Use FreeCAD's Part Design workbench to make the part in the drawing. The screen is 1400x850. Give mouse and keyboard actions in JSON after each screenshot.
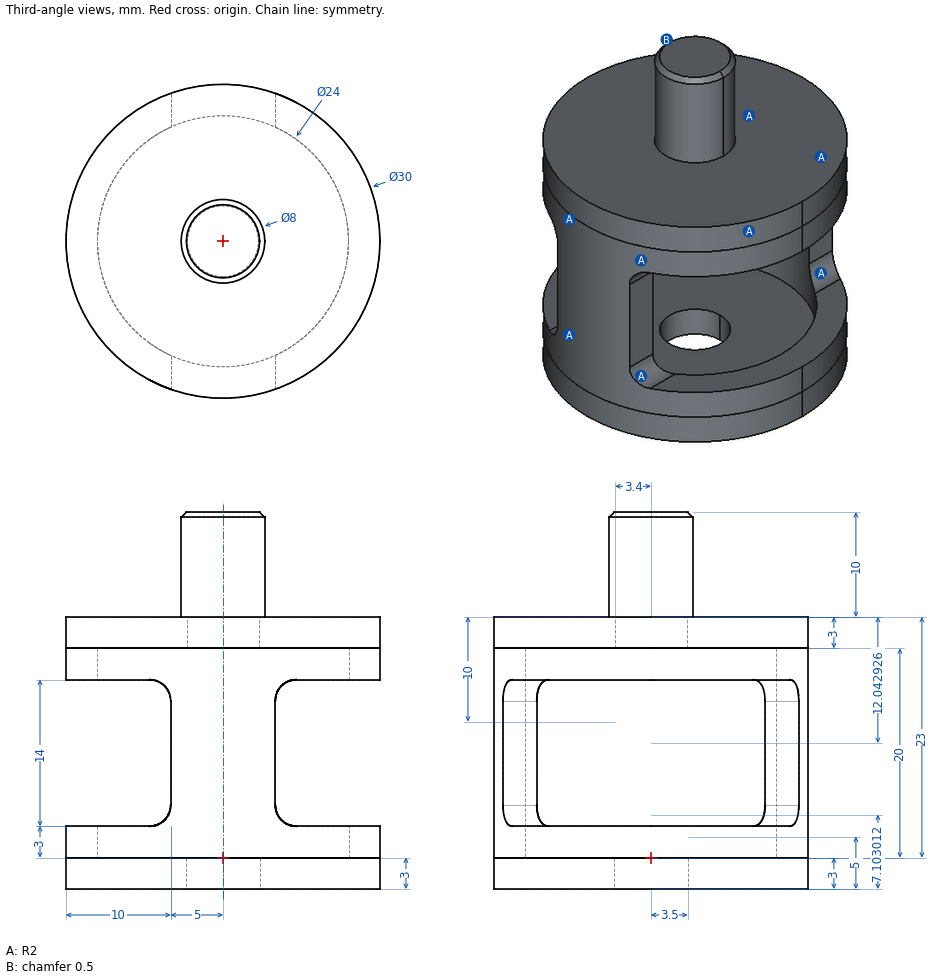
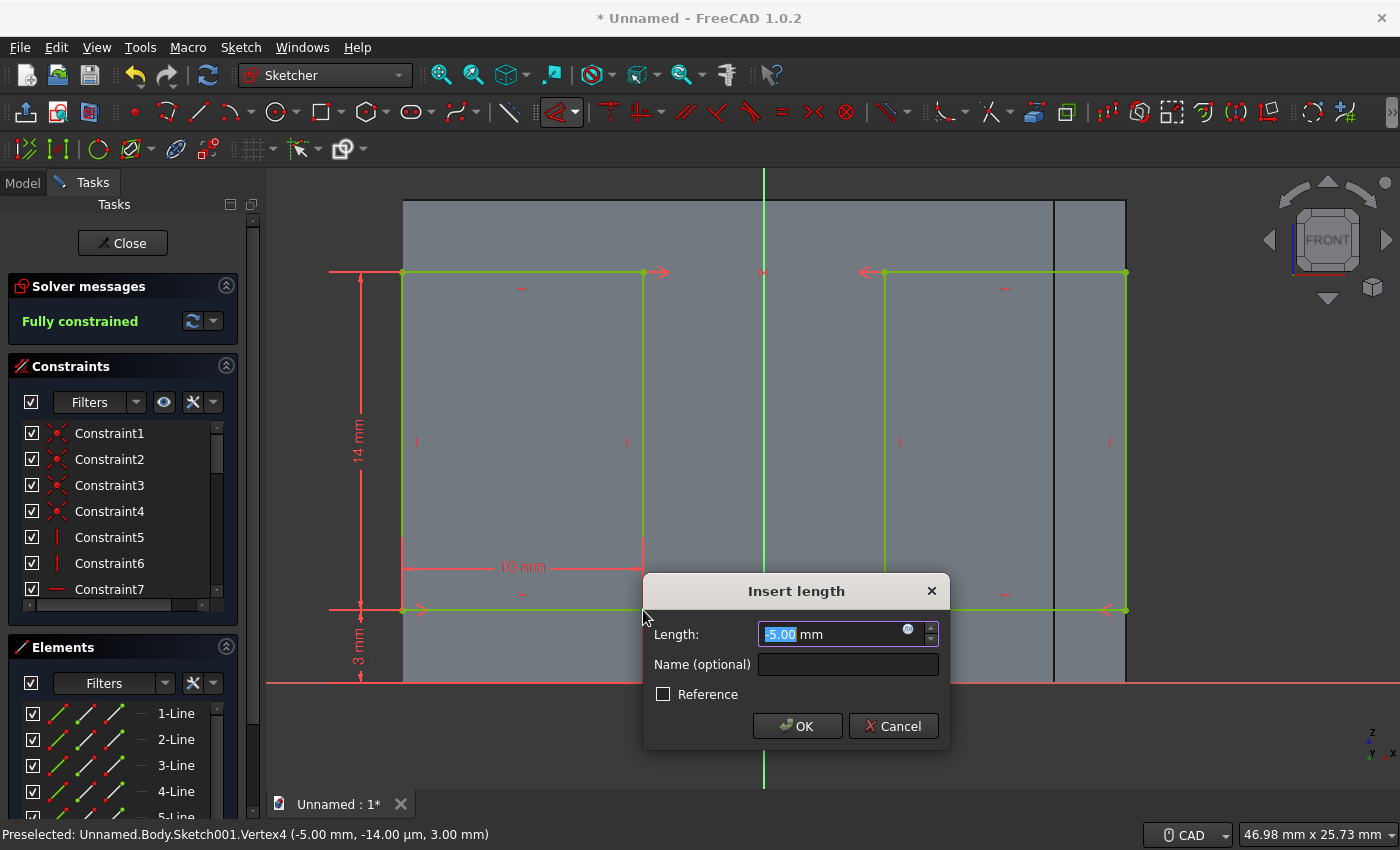
{"action": "type", "text": "-5"}
{"action": "key", "text": "Return"}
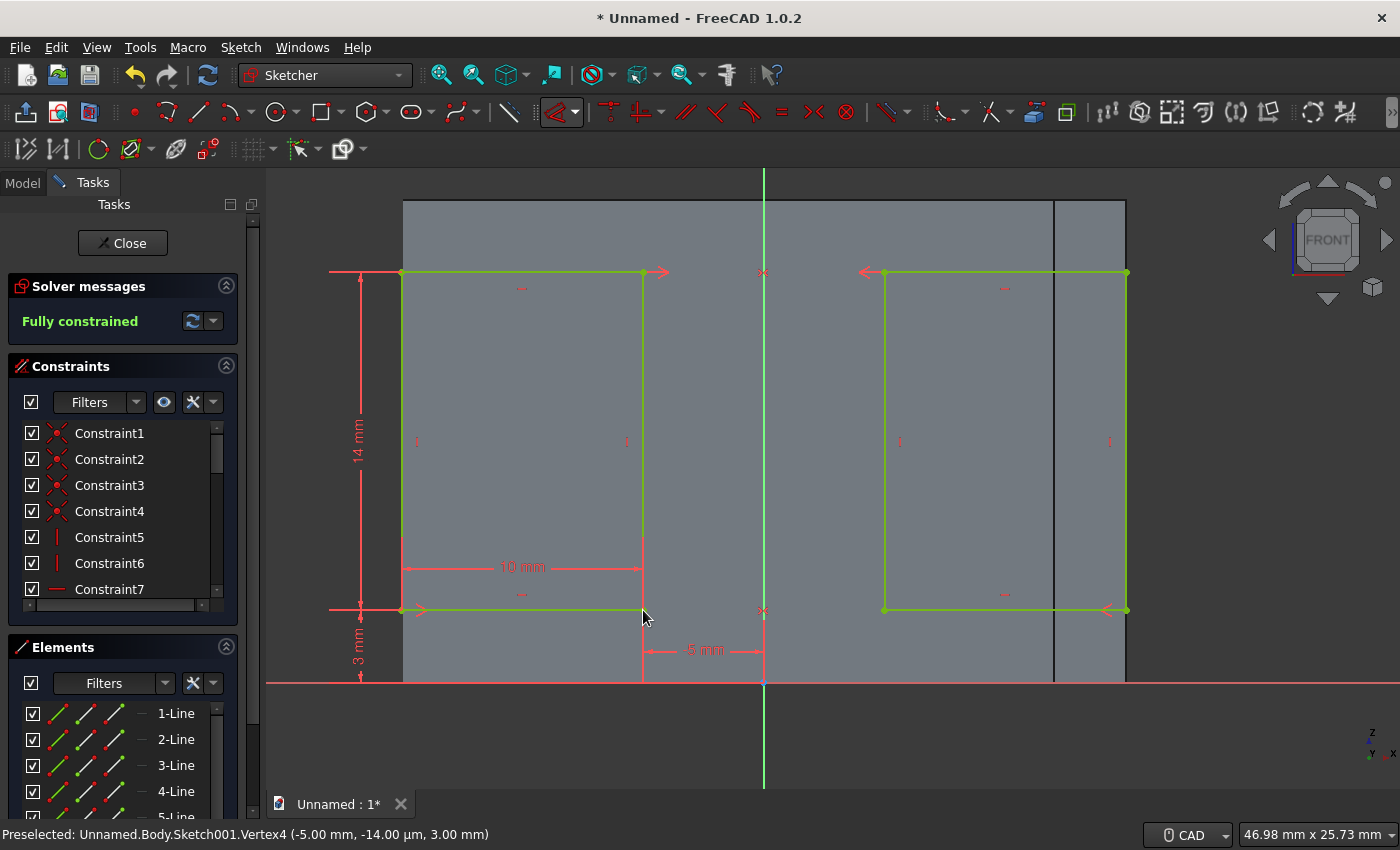
{"action": "left_click", "coordinate": [123, 243]}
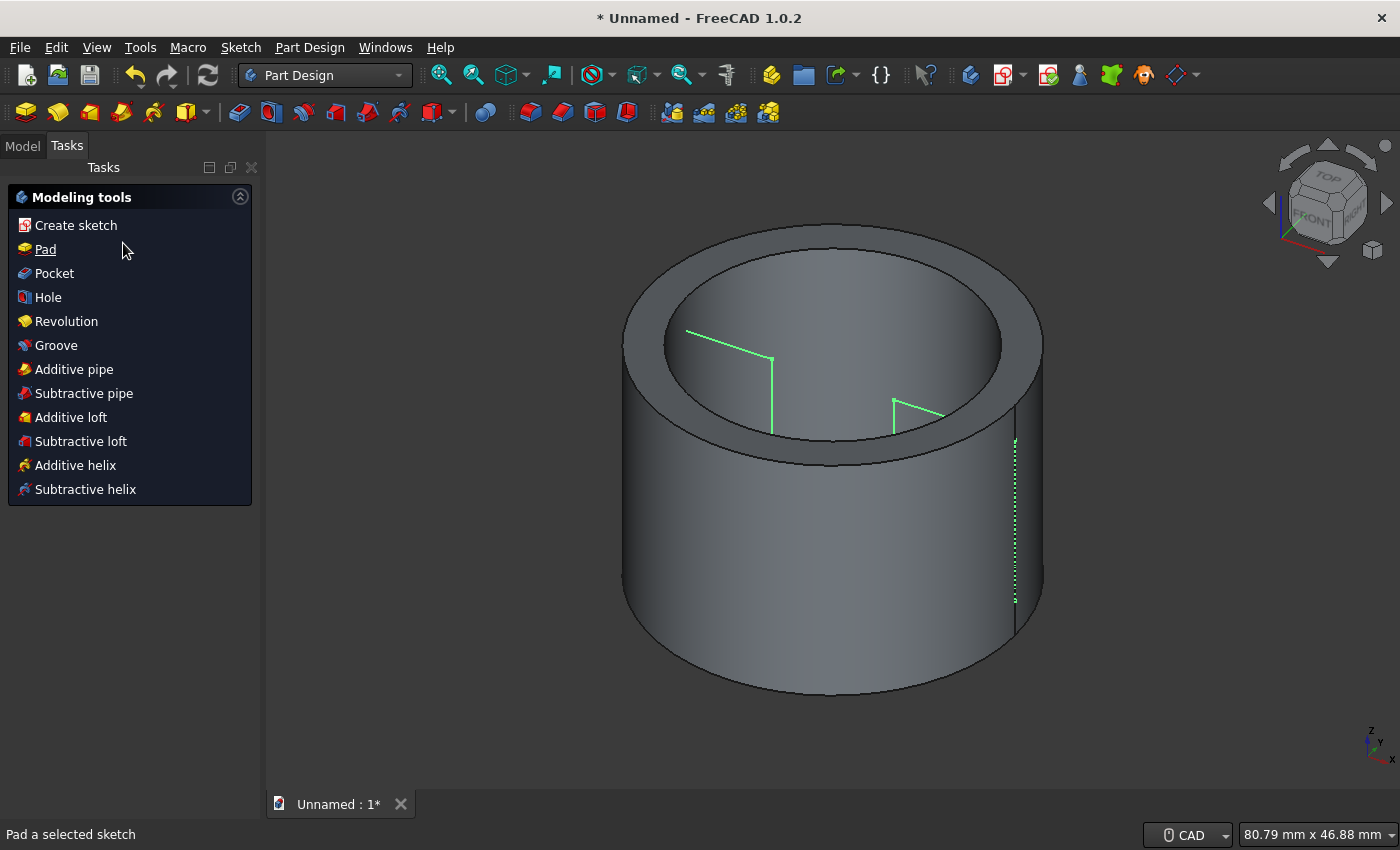
{"action": "left_click", "coordinate": [240, 112]}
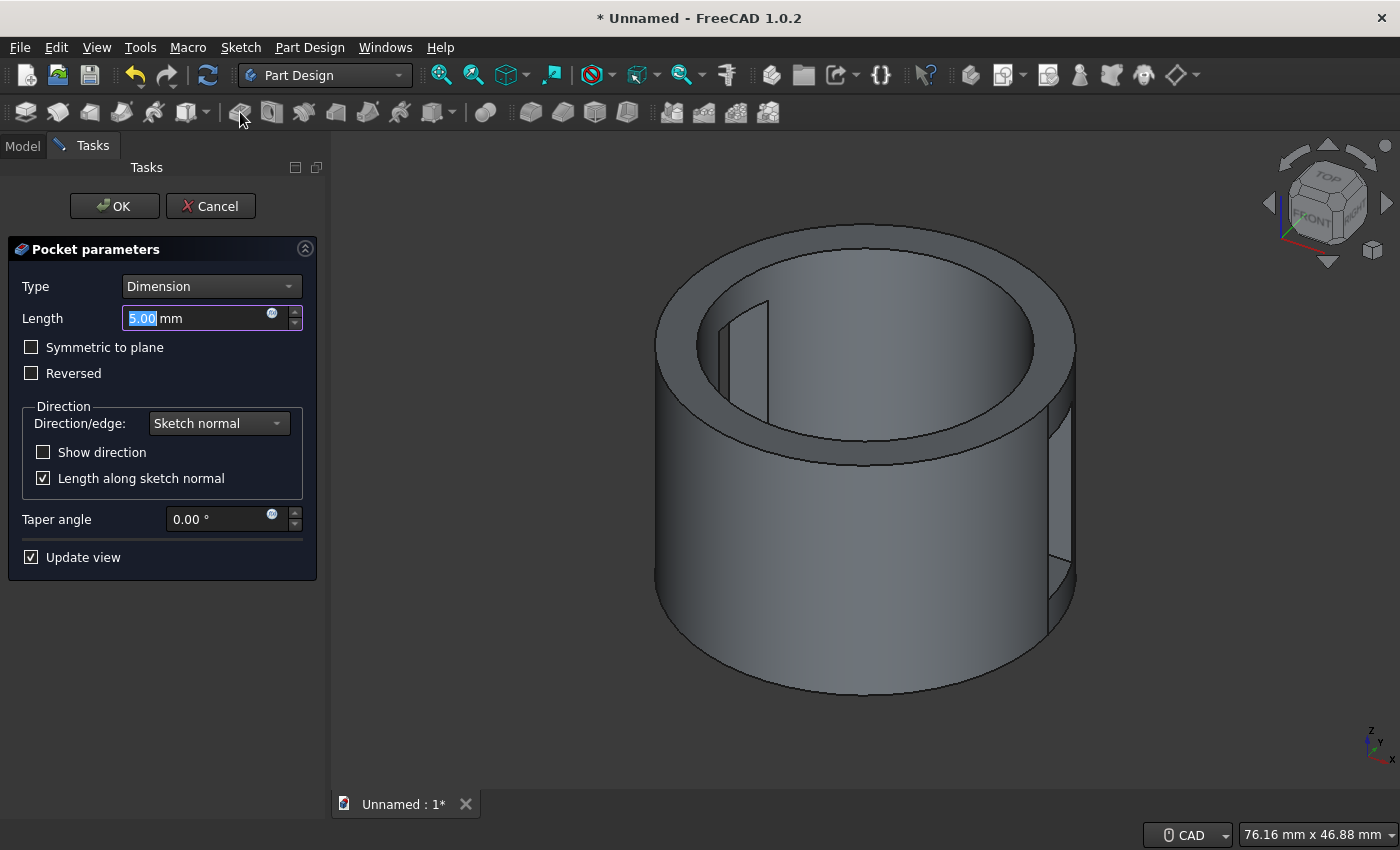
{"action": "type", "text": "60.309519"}
{"action": "key", "text": "Tab"}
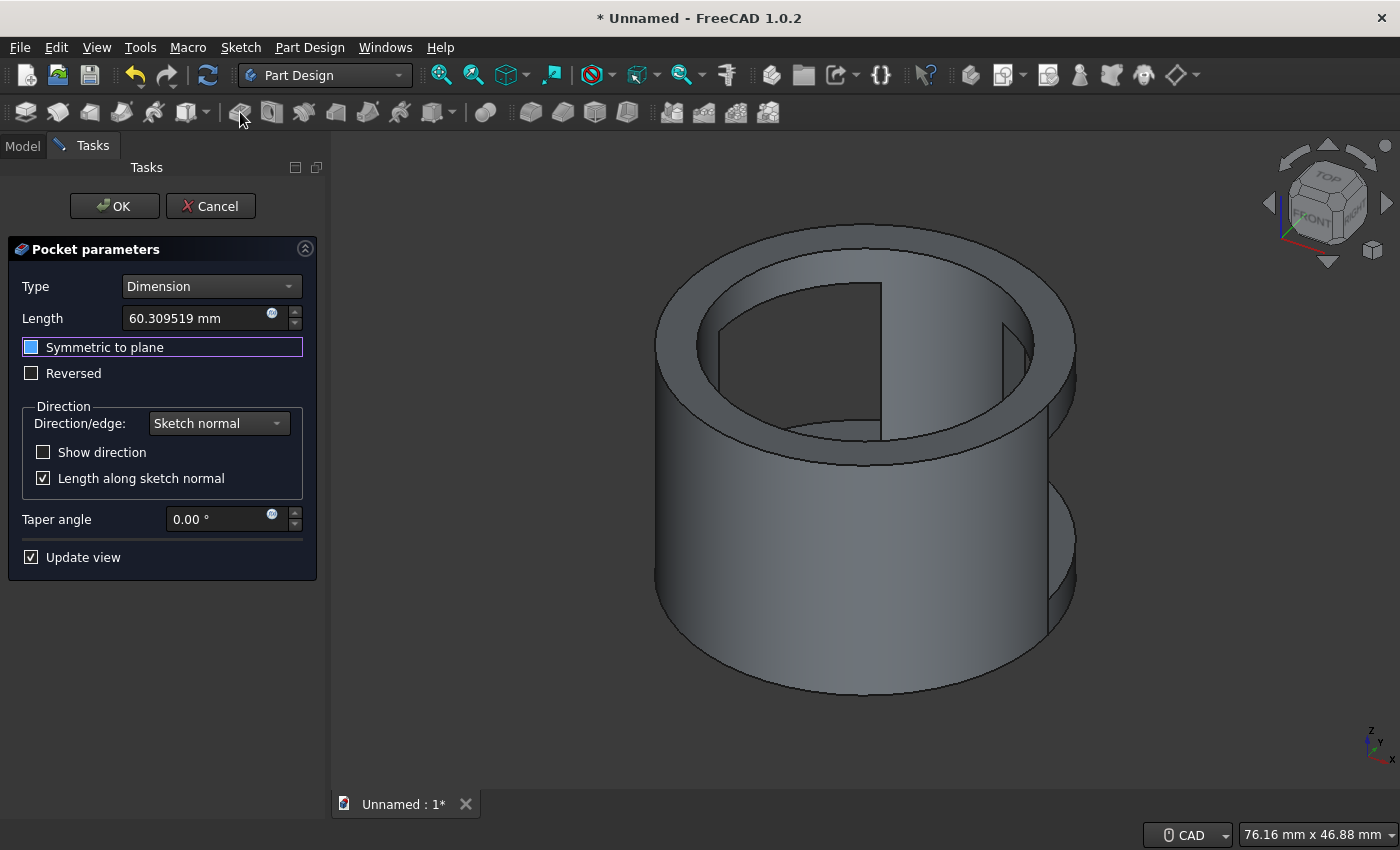
{"action": "left_click", "coordinate": [30, 347]}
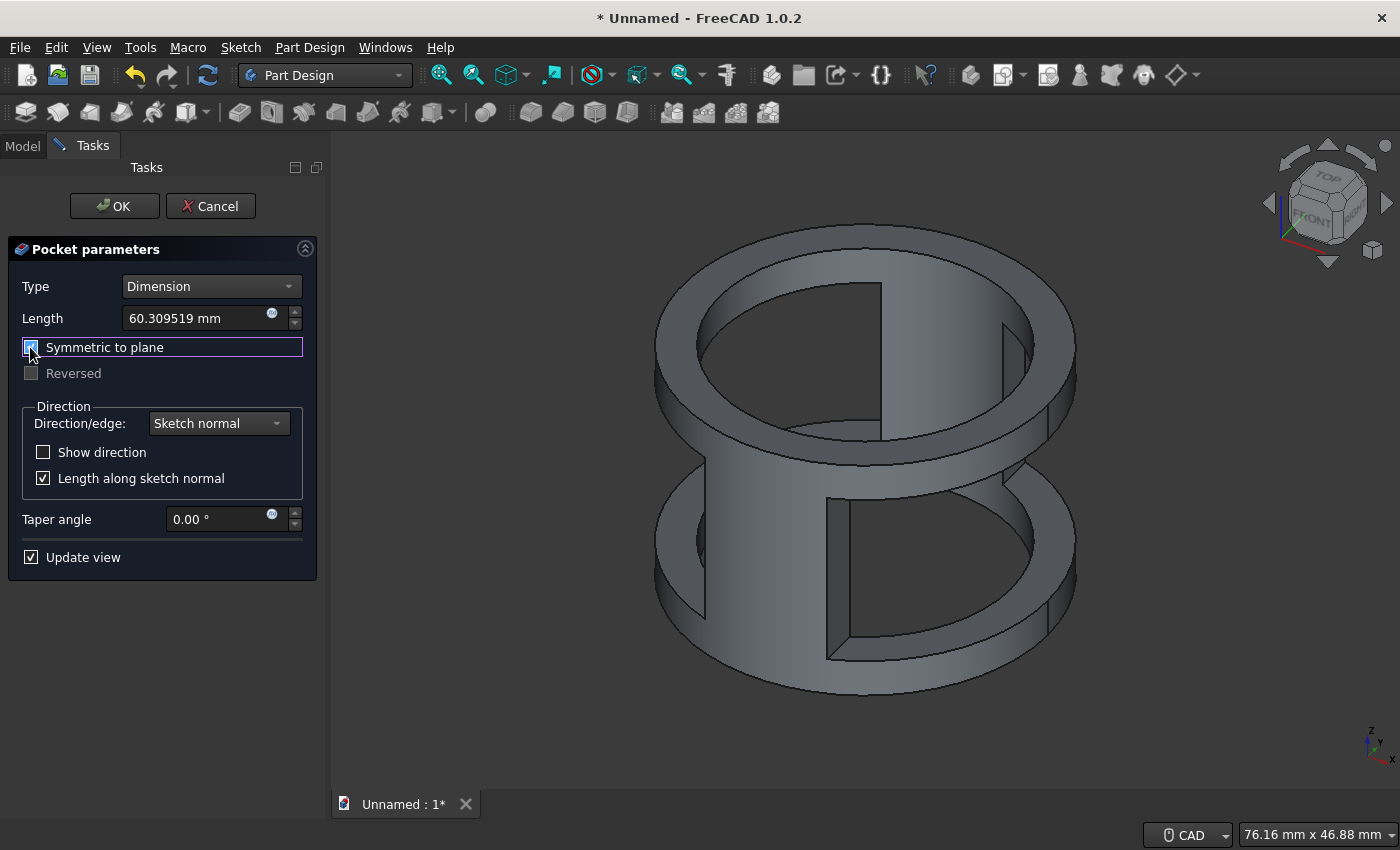
{"action": "left_click", "coordinate": [115, 206]}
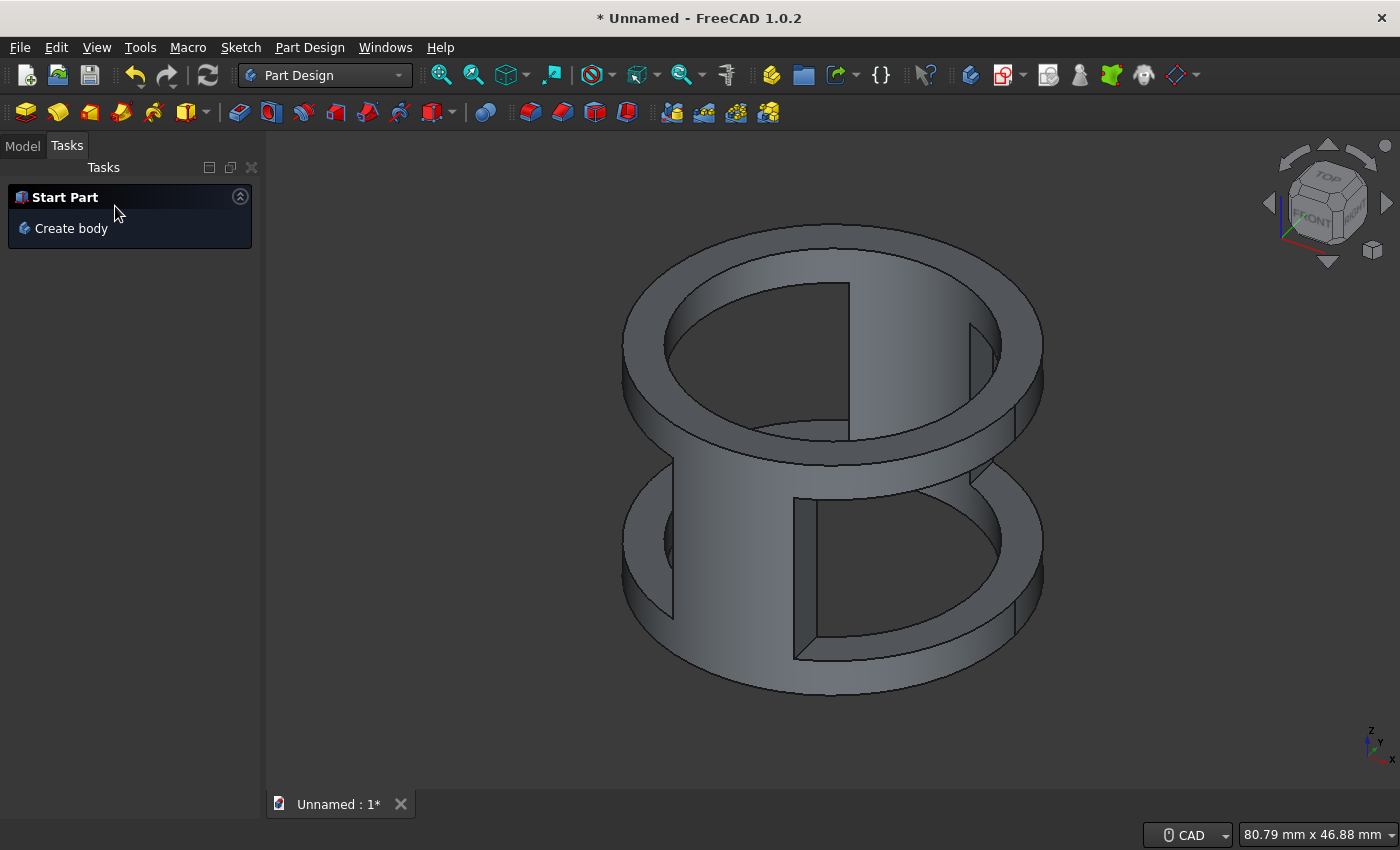
{"action": "key", "text": "0"}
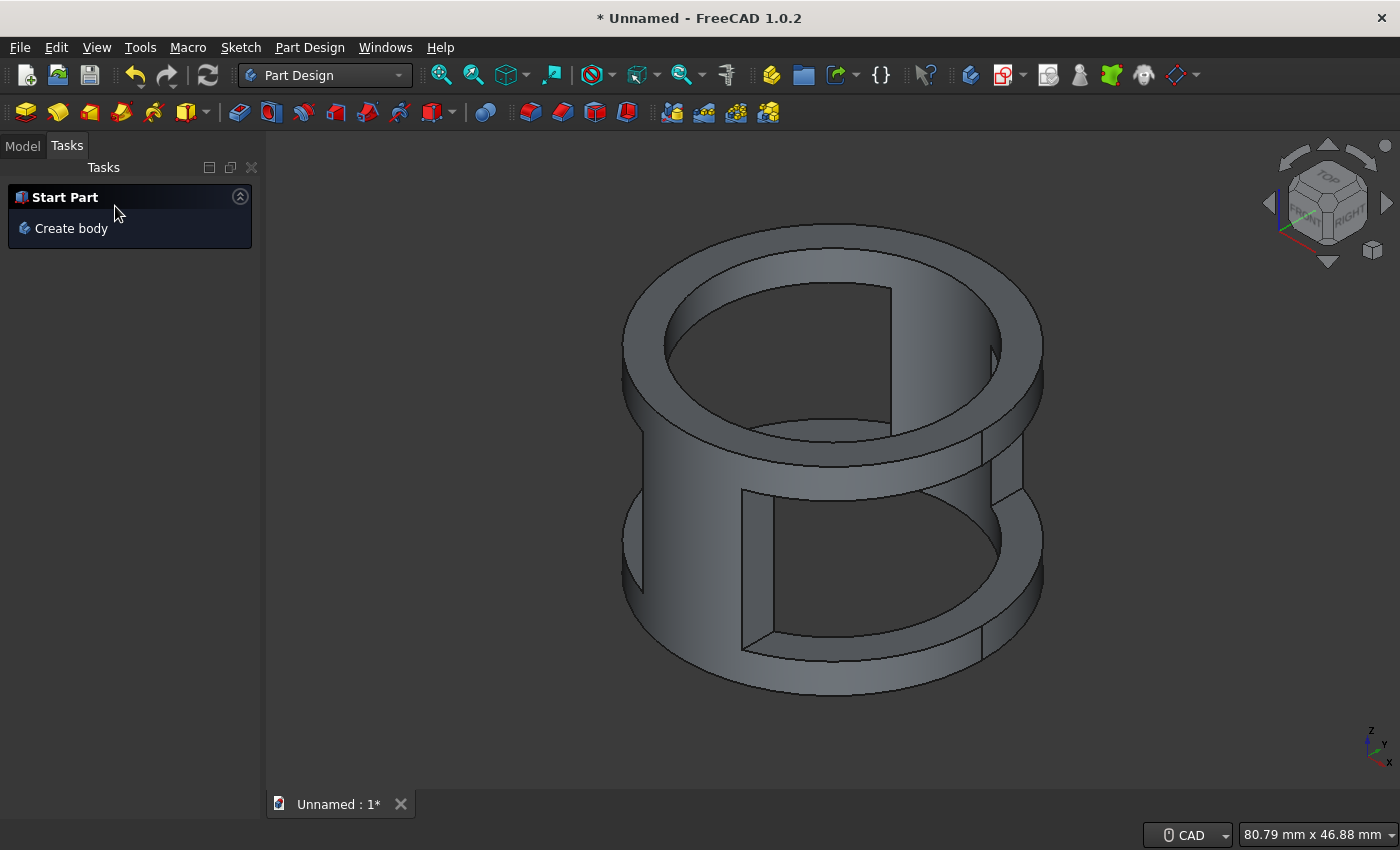
{"action": "key", "text": "2"}